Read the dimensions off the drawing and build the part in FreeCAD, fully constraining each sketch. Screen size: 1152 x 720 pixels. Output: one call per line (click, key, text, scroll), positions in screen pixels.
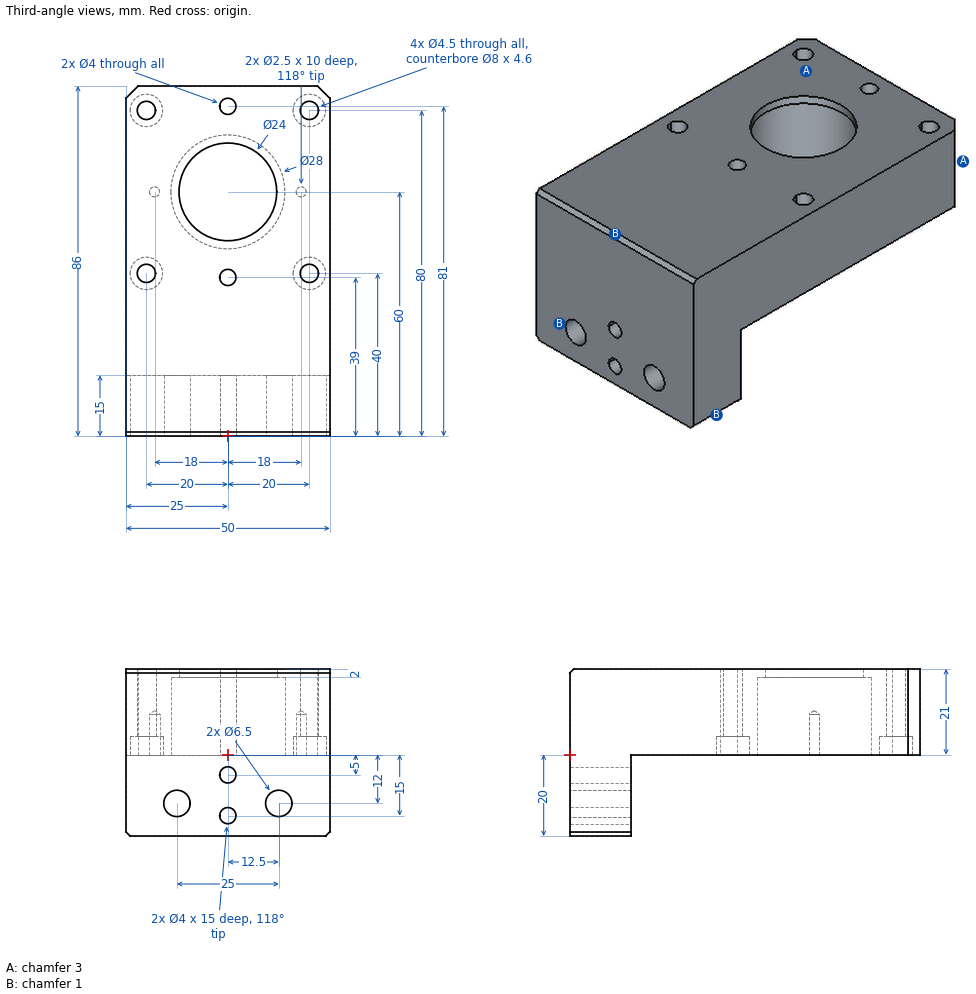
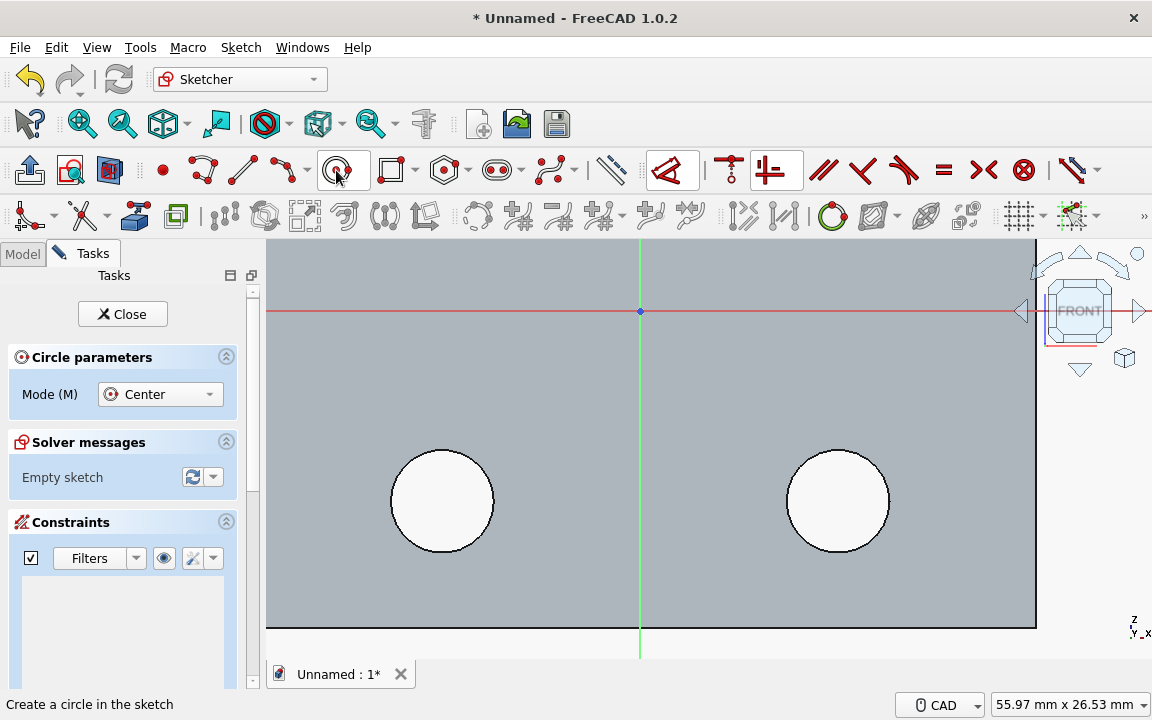
click(640, 549)
click(663, 527)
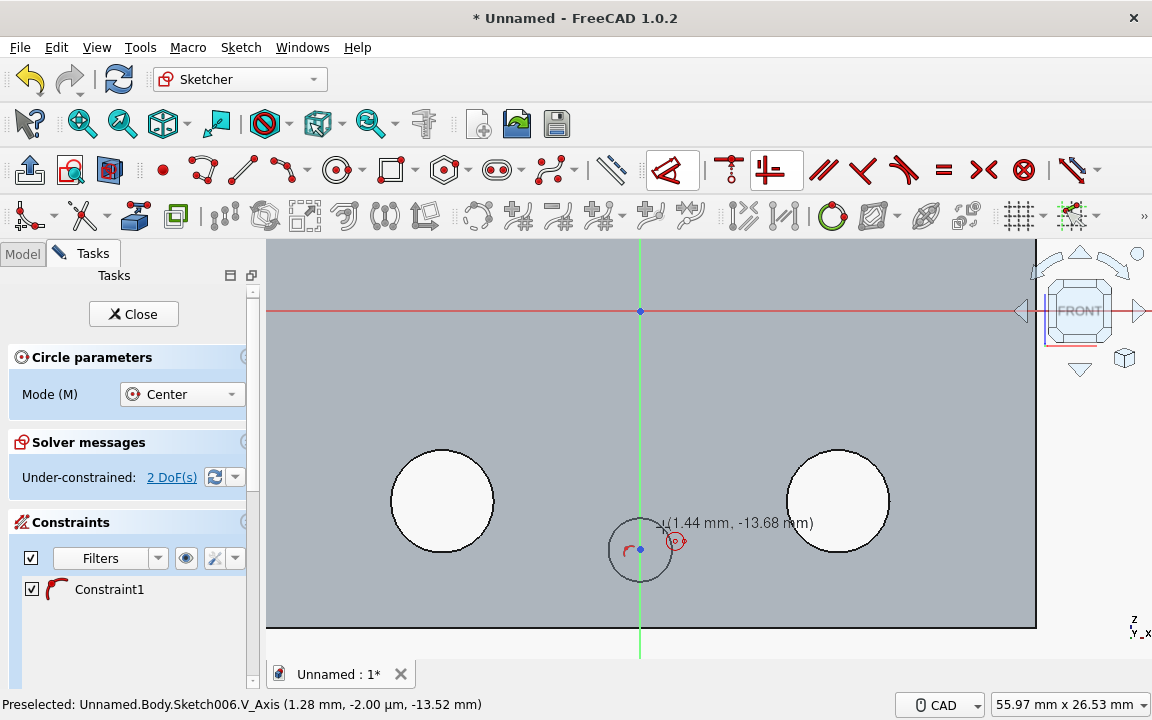
click(640, 391)
click(663, 368)
key(Escape)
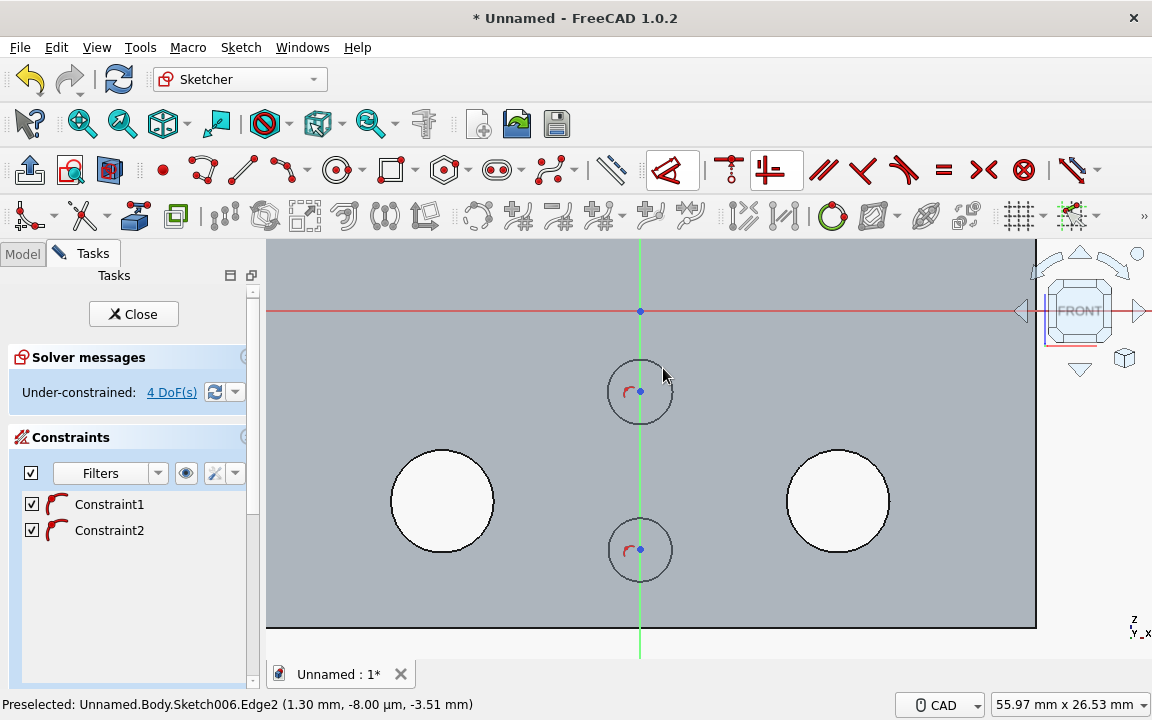
click(663, 528)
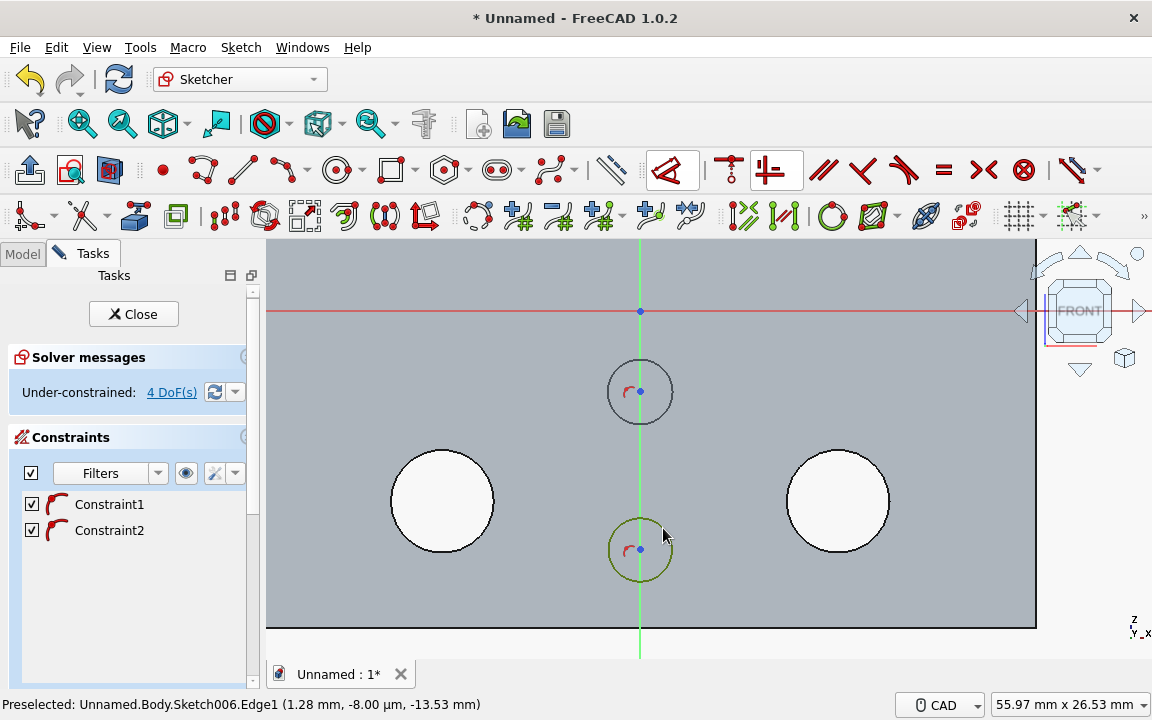
click(663, 369)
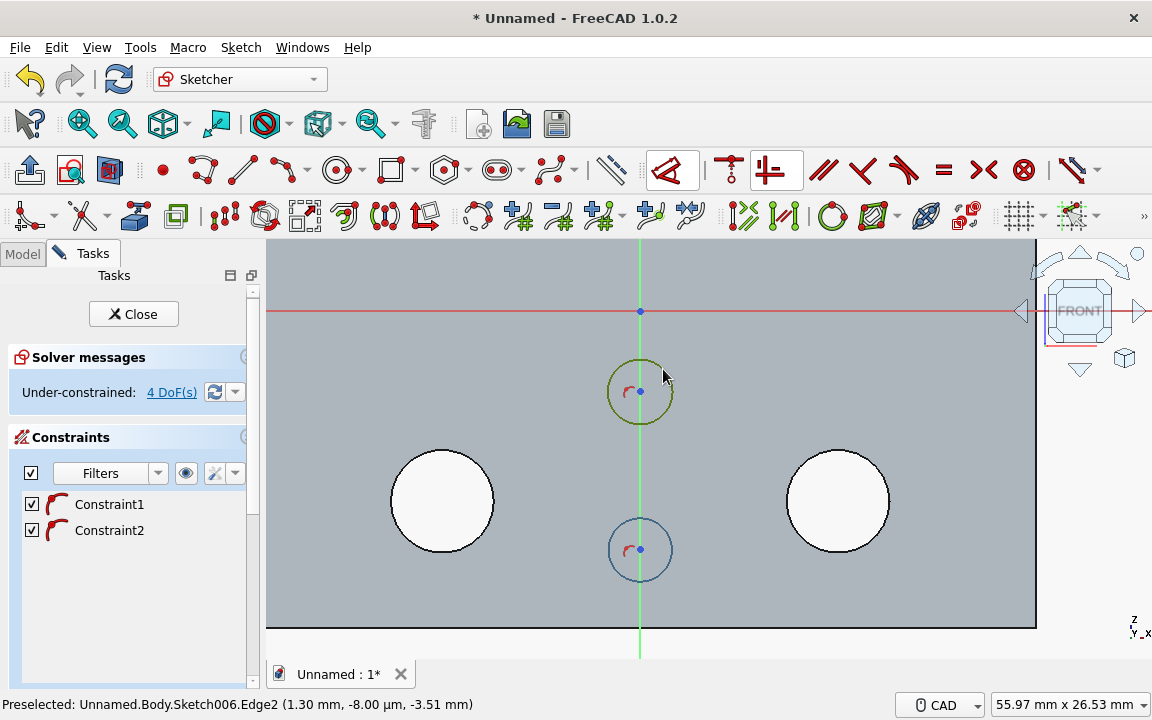
click(944, 170)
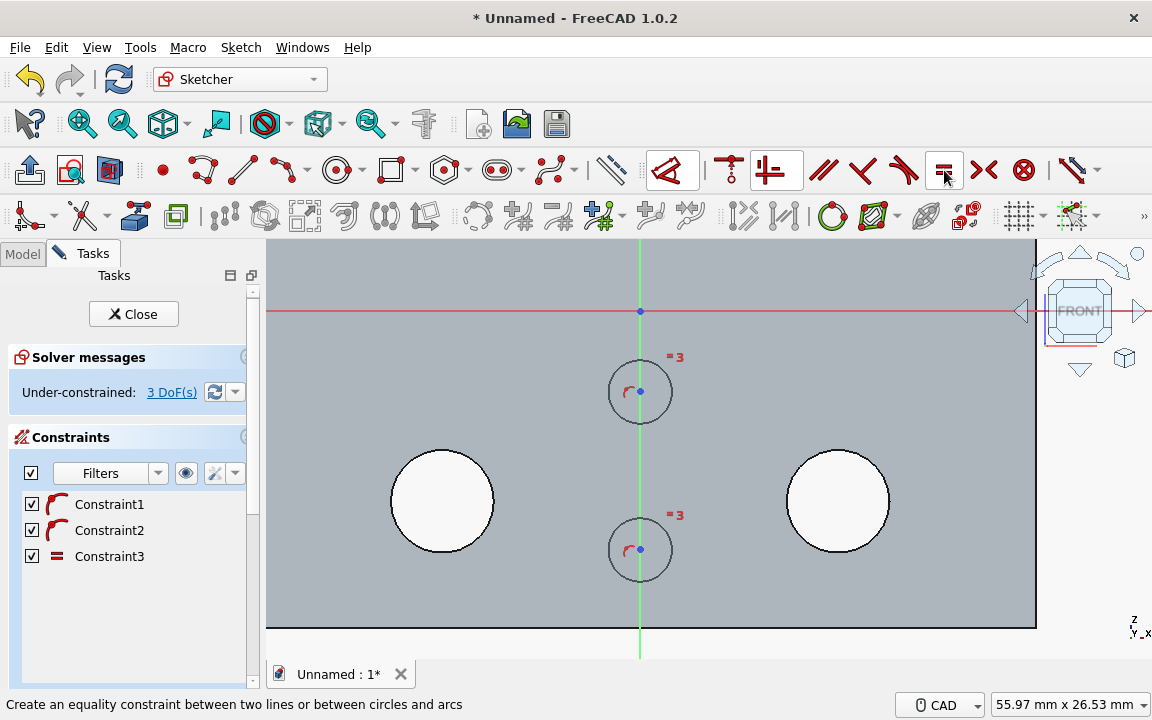
click(663, 528)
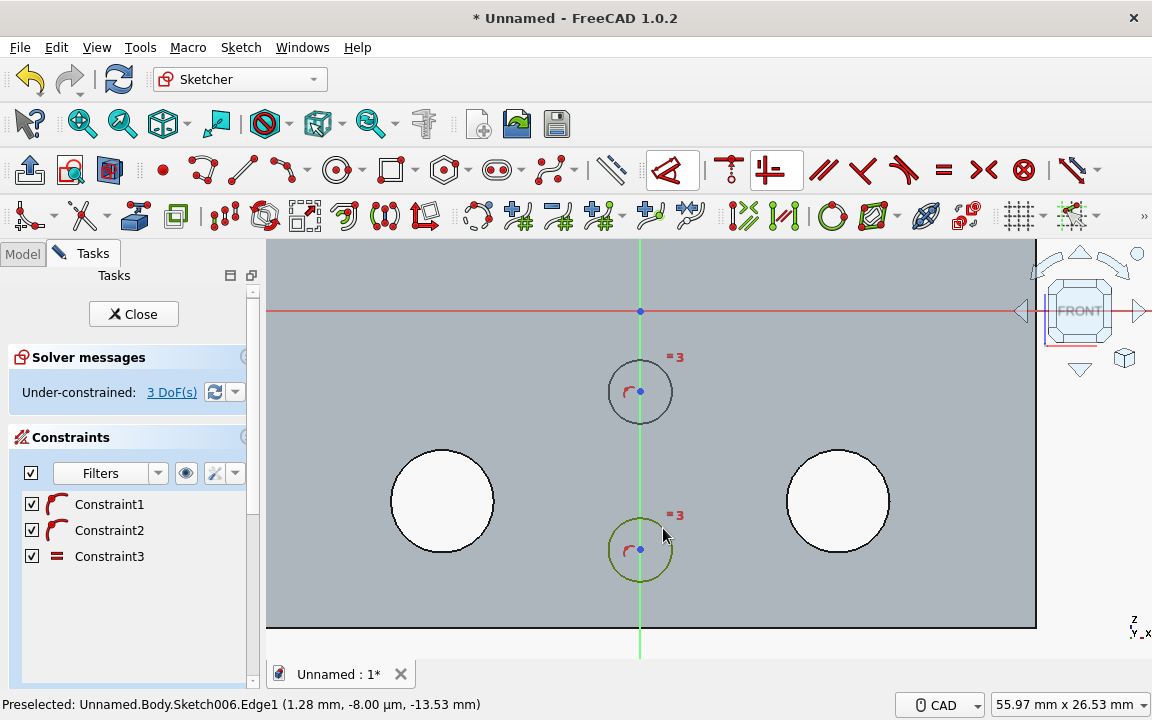
key(k)
key(o)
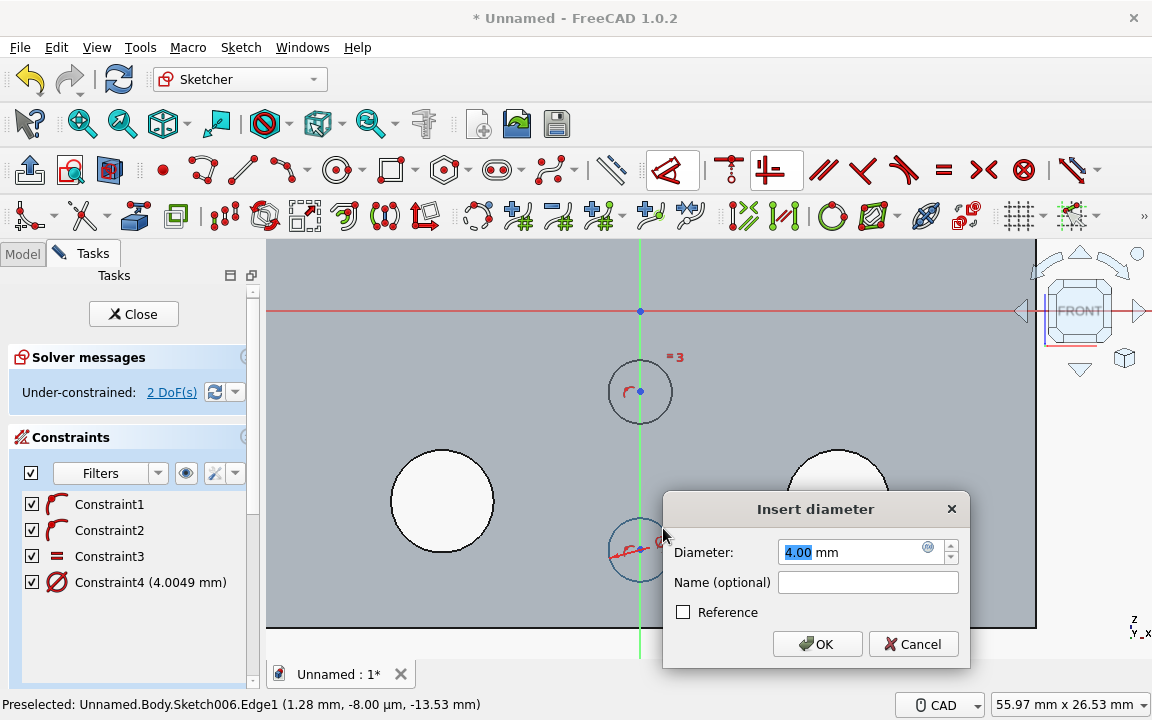
text(4)
key(Return)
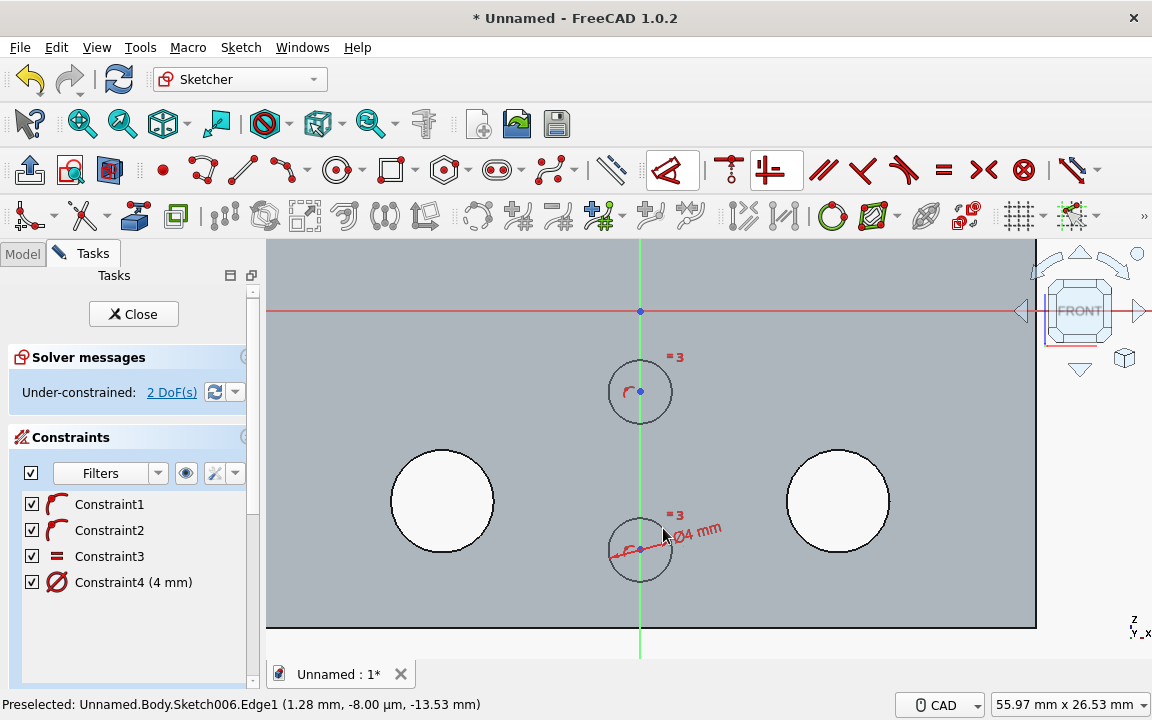
click(640, 392)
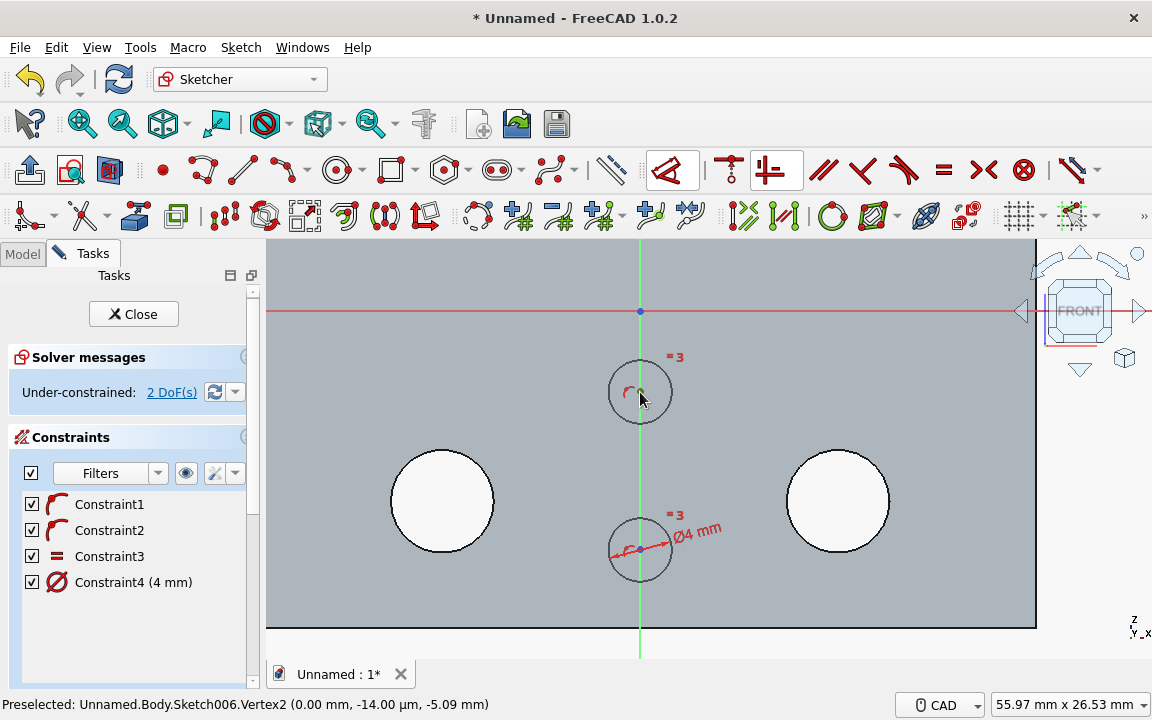
click(694, 170)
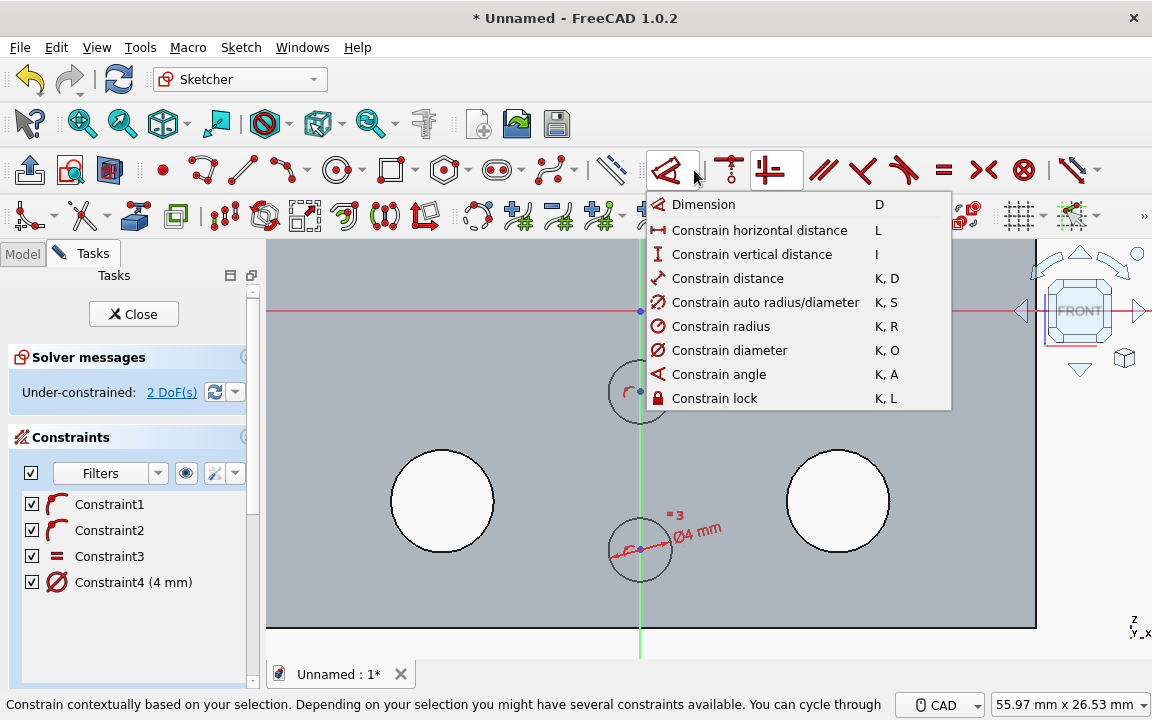
click(799, 254)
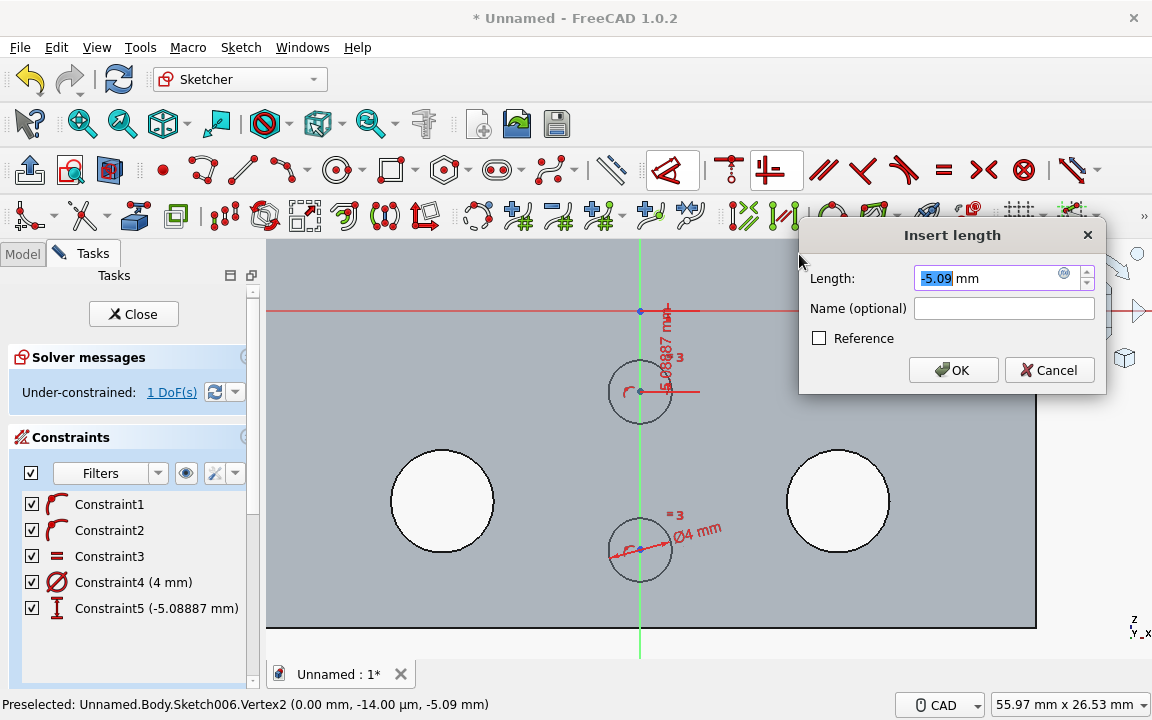
text(-5)
key(Return)